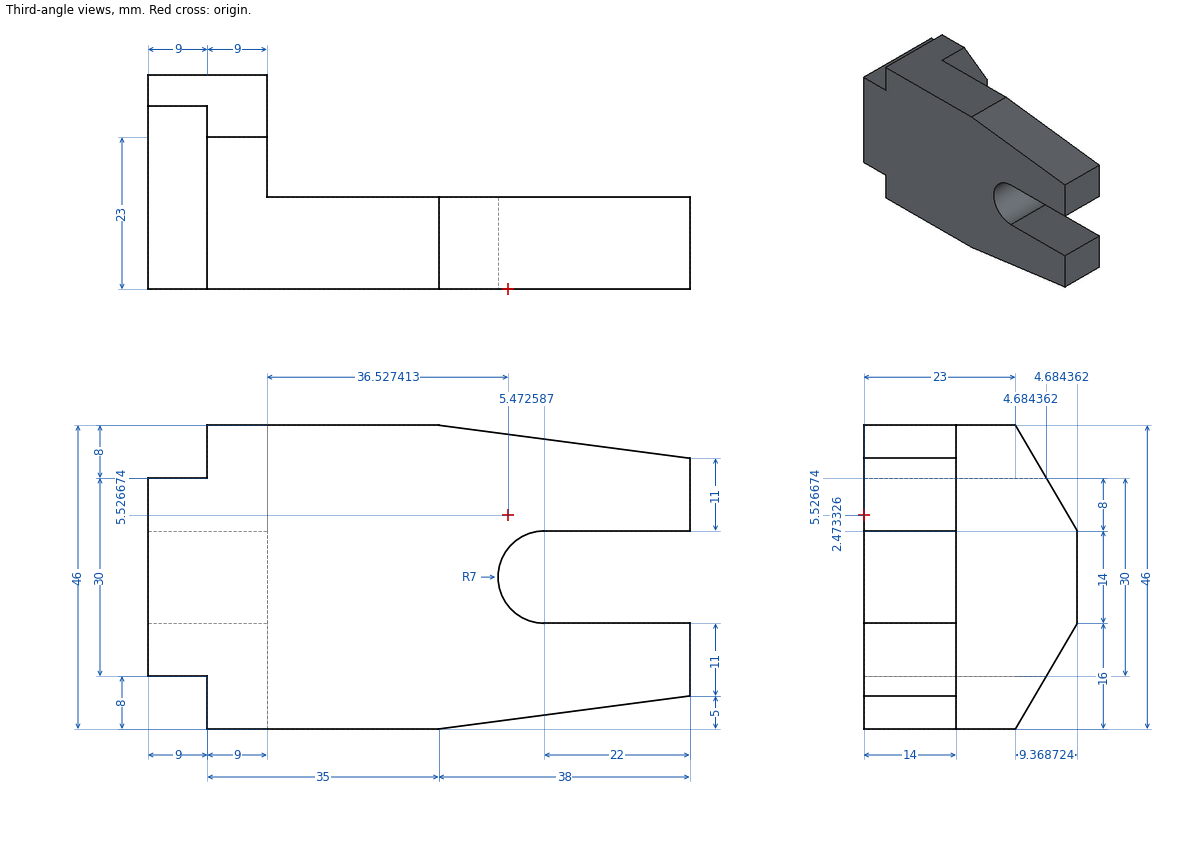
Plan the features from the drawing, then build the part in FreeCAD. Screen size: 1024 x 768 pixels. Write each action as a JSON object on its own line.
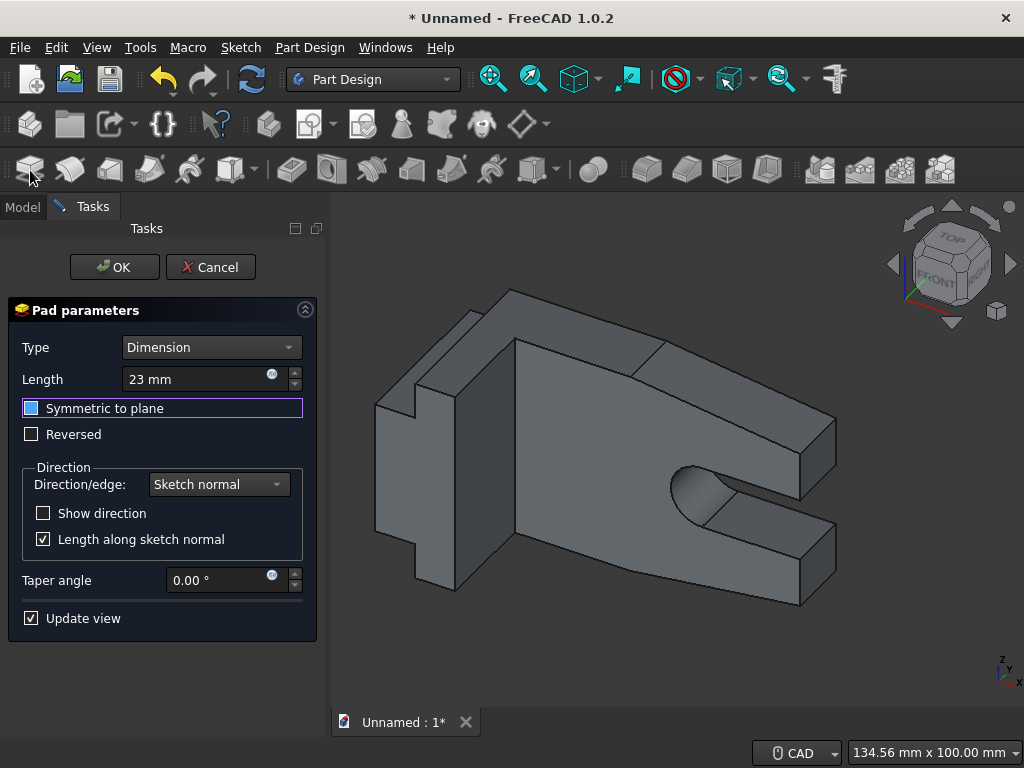
{"action": "left_click", "coordinate": [30, 434]}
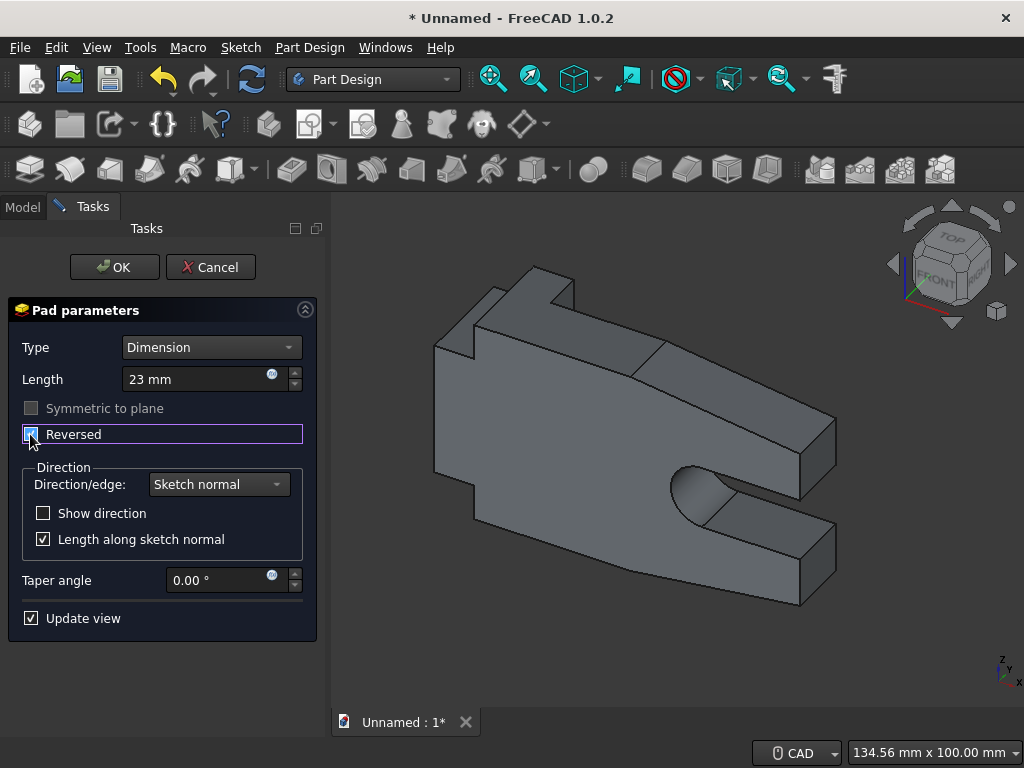
{"action": "left_click", "coordinate": [115, 267]}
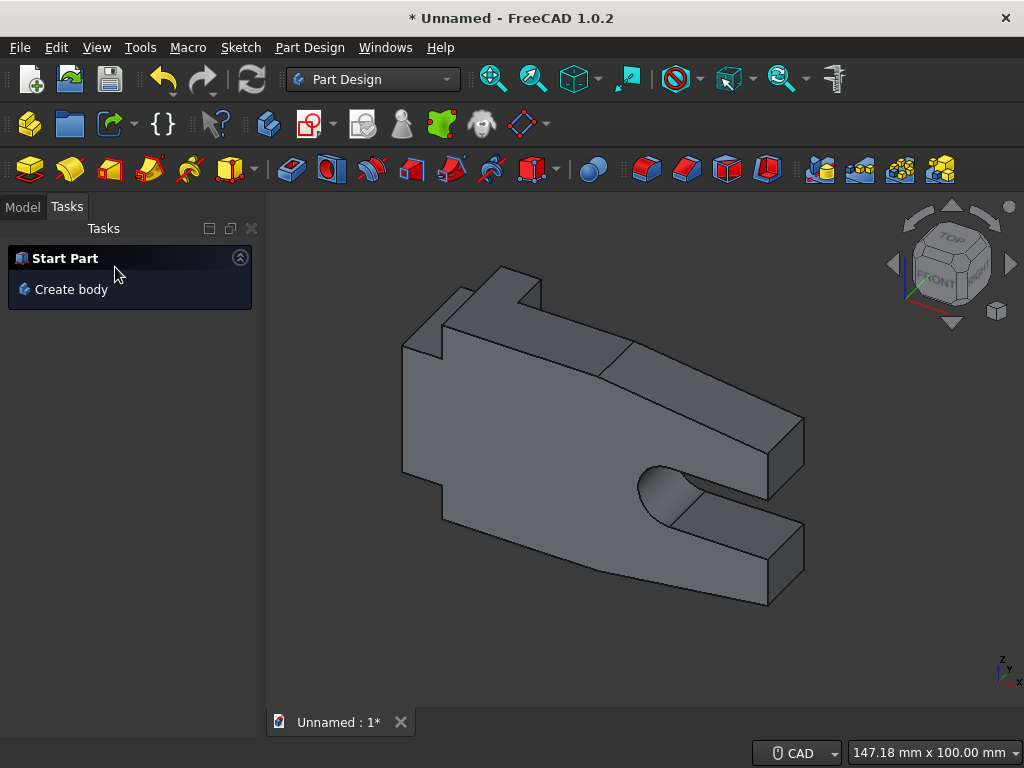
{"action": "key", "text": "0"}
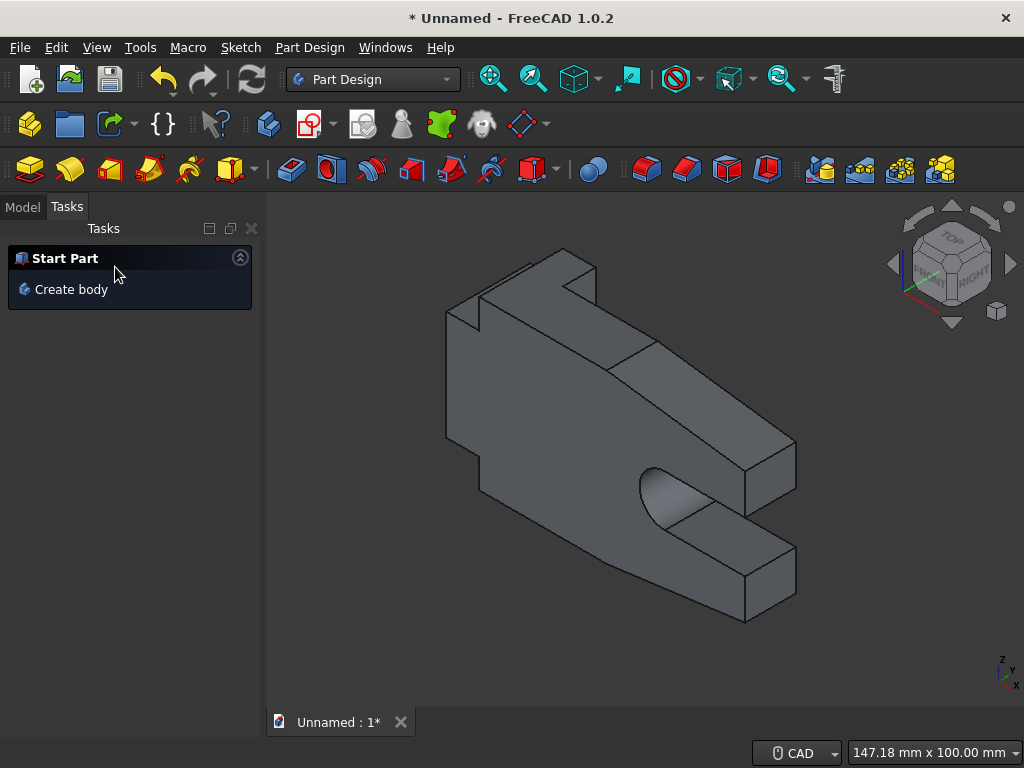
{"action": "key", "text": "3"}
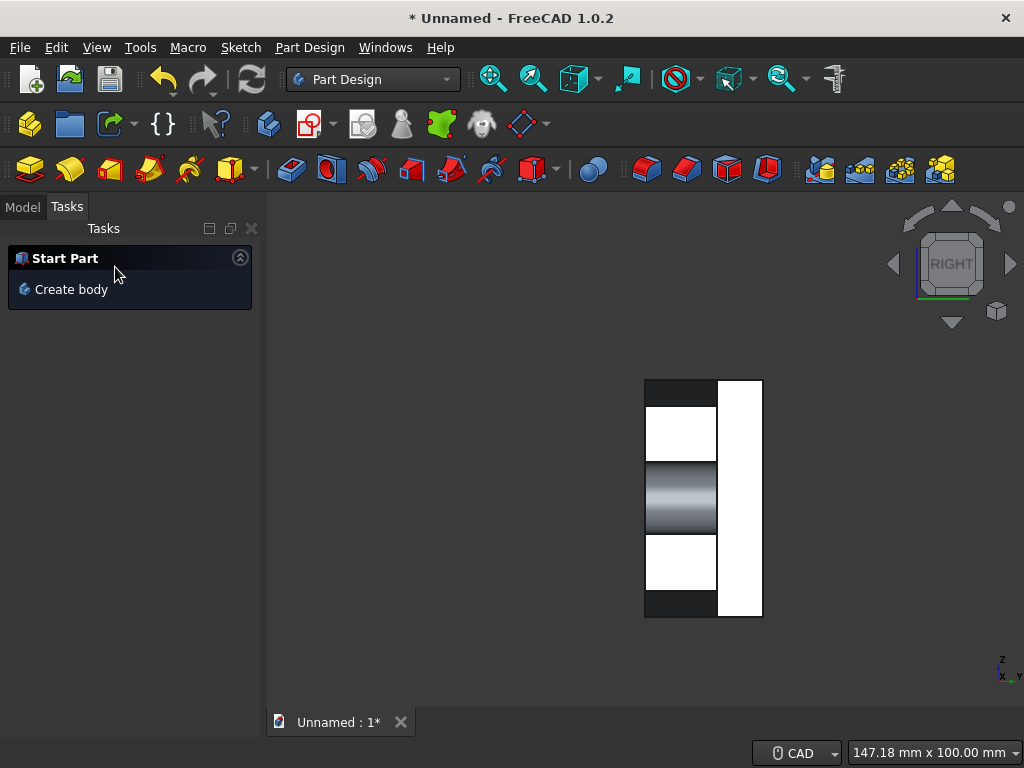
{"action": "left_click", "coordinate": [740, 463]}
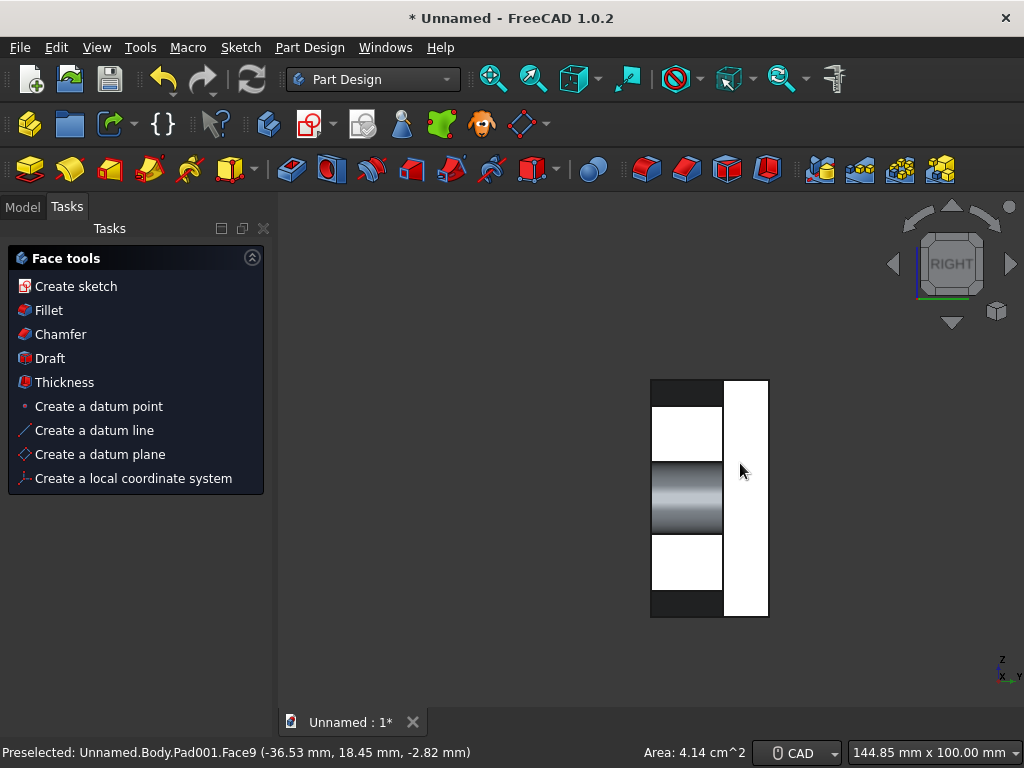
{"action": "left_click", "coordinate": [310, 124]}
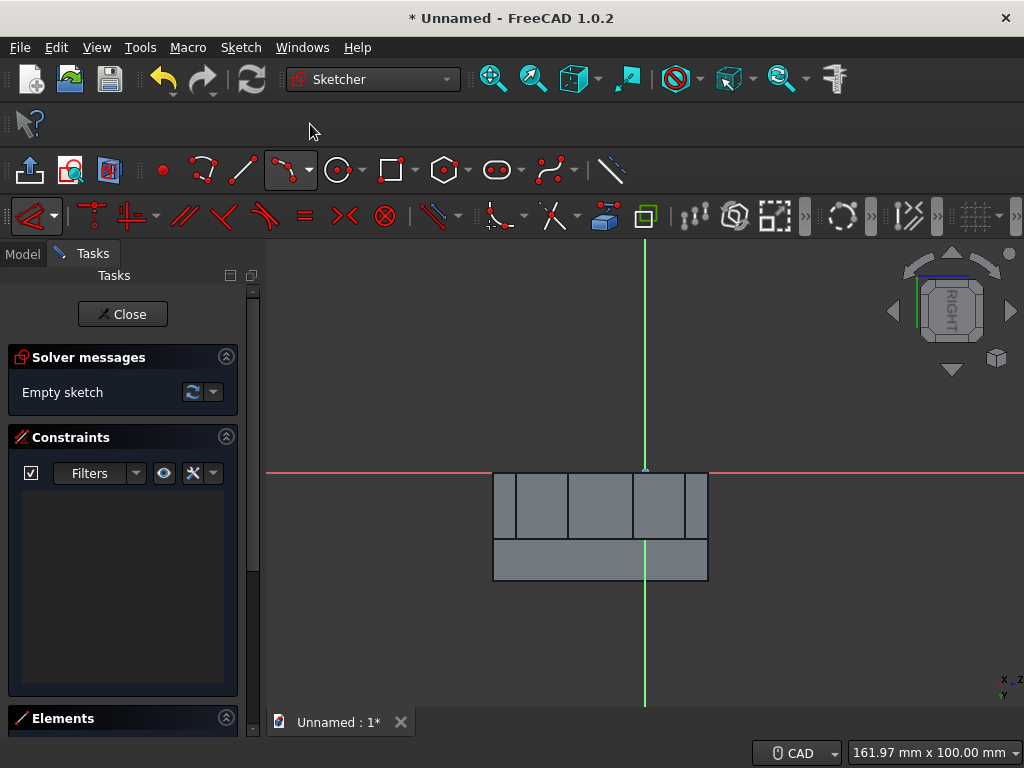
{"action": "left_click", "coordinate": [110, 170]}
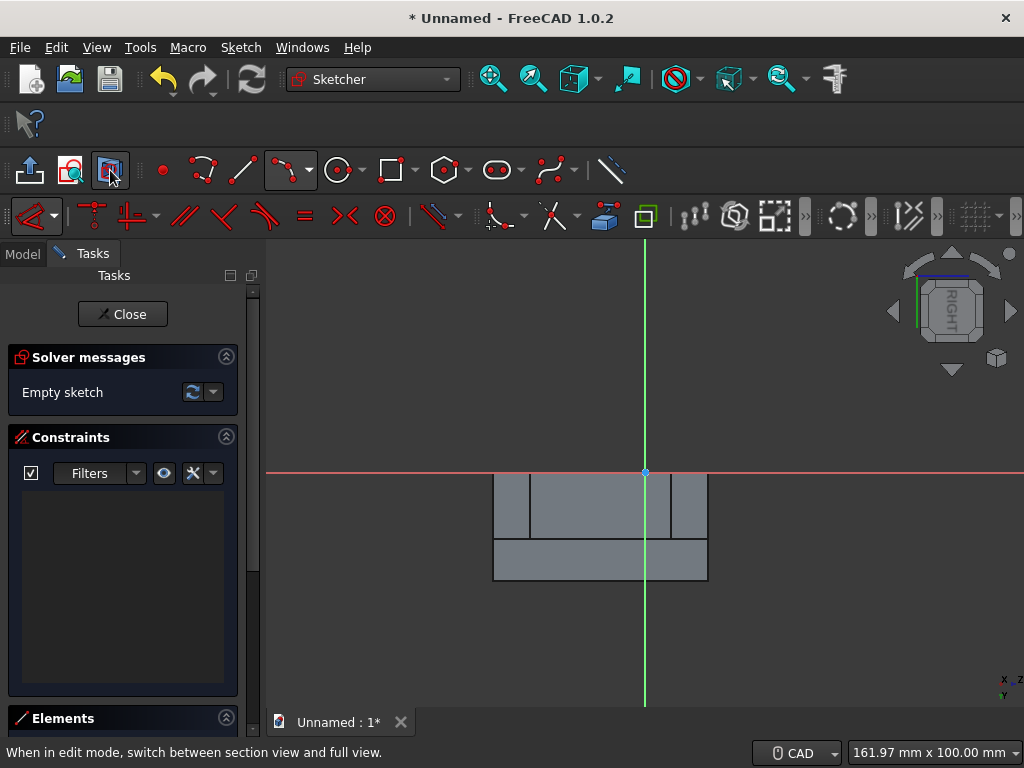
{"action": "scroll", "coordinate": [630, 641], "scroll_direction": "up", "scroll_amount": 3}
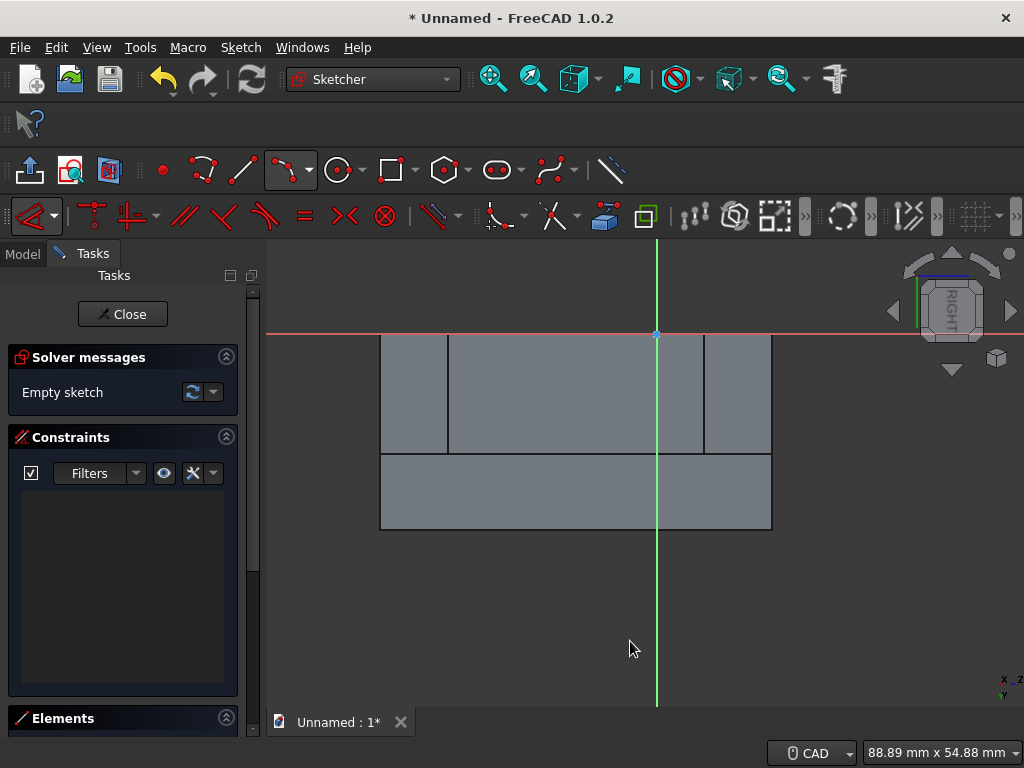
{"action": "left_click", "coordinate": [204, 170]}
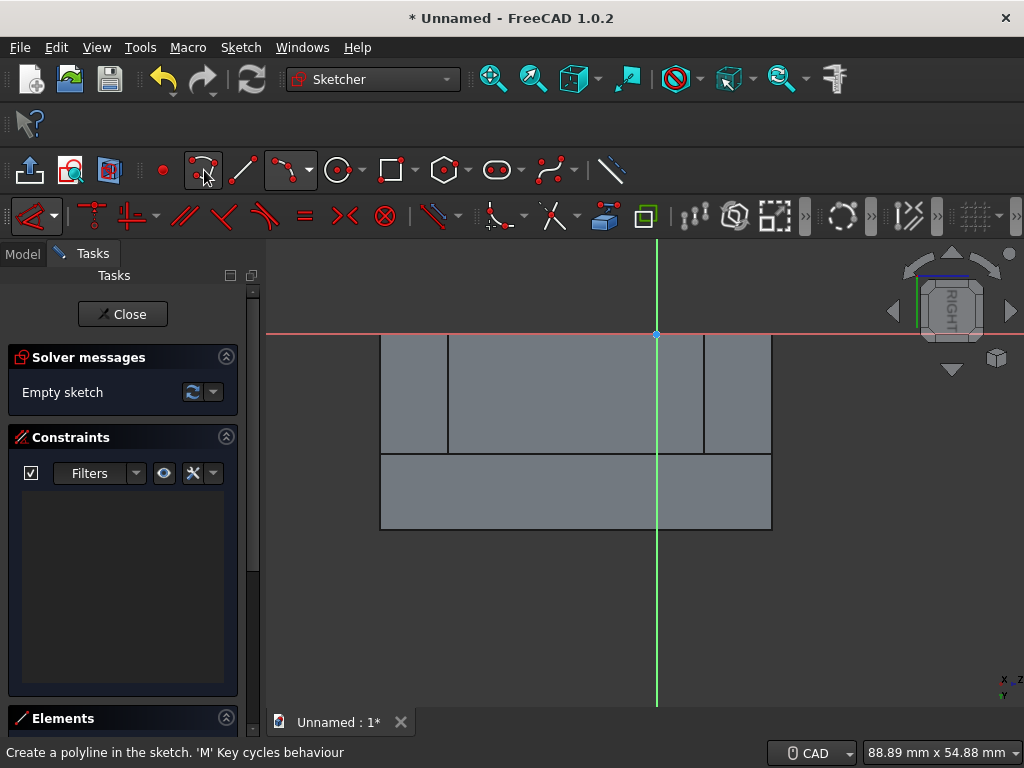
{"action": "left_click", "coordinate": [772, 530]}
{"action": "left_click", "coordinate": [380, 530]}
{"action": "left_click", "coordinate": [516, 610]}
{"action": "left_click", "coordinate": [636, 610]}
{"action": "left_click", "coordinate": [772, 531]}
{"action": "key", "text": "Escape"}
{"action": "key", "text": "Escape"}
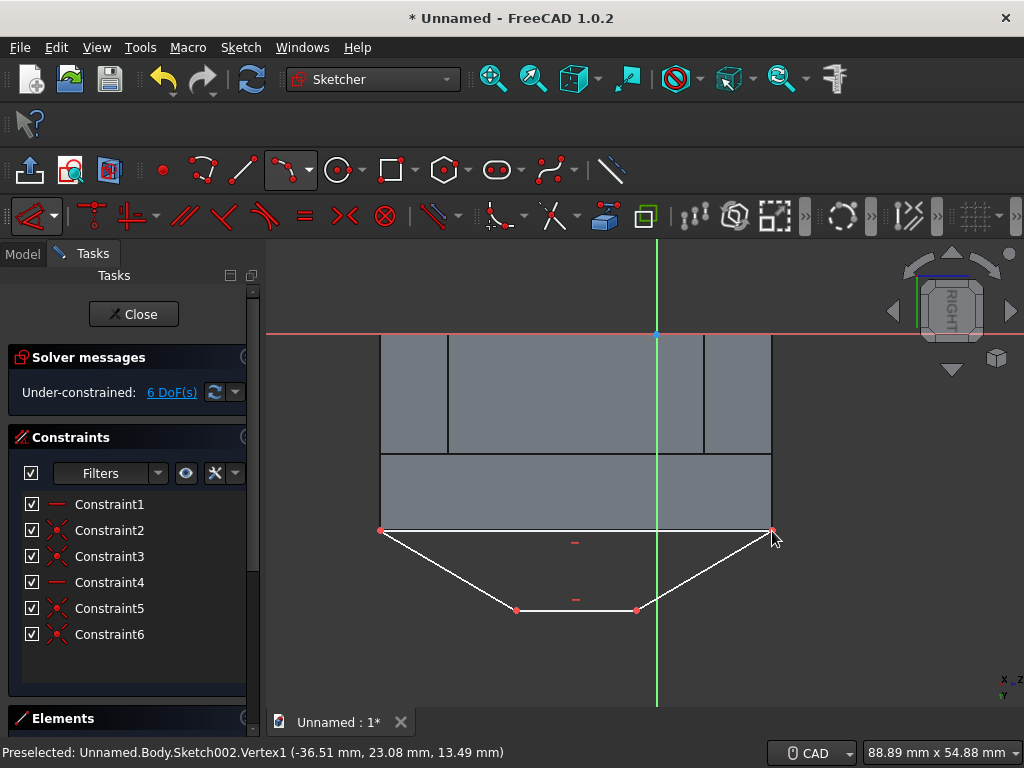
{"action": "left_click", "coordinate": [654, 531]}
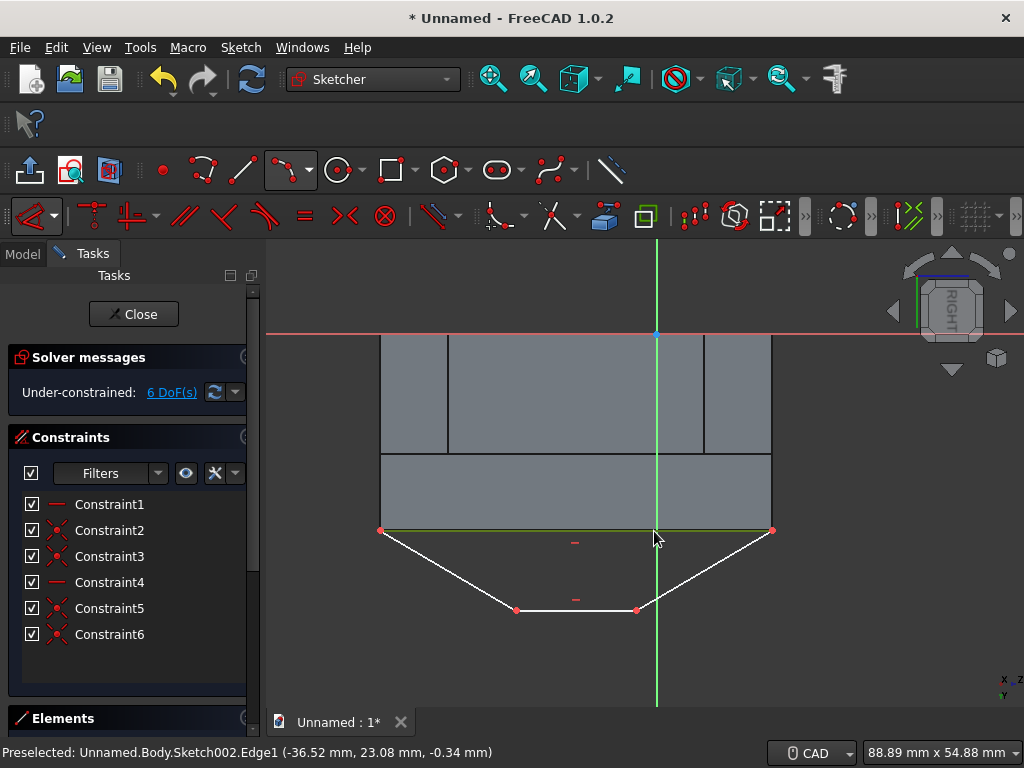
{"action": "key", "text": "l"}